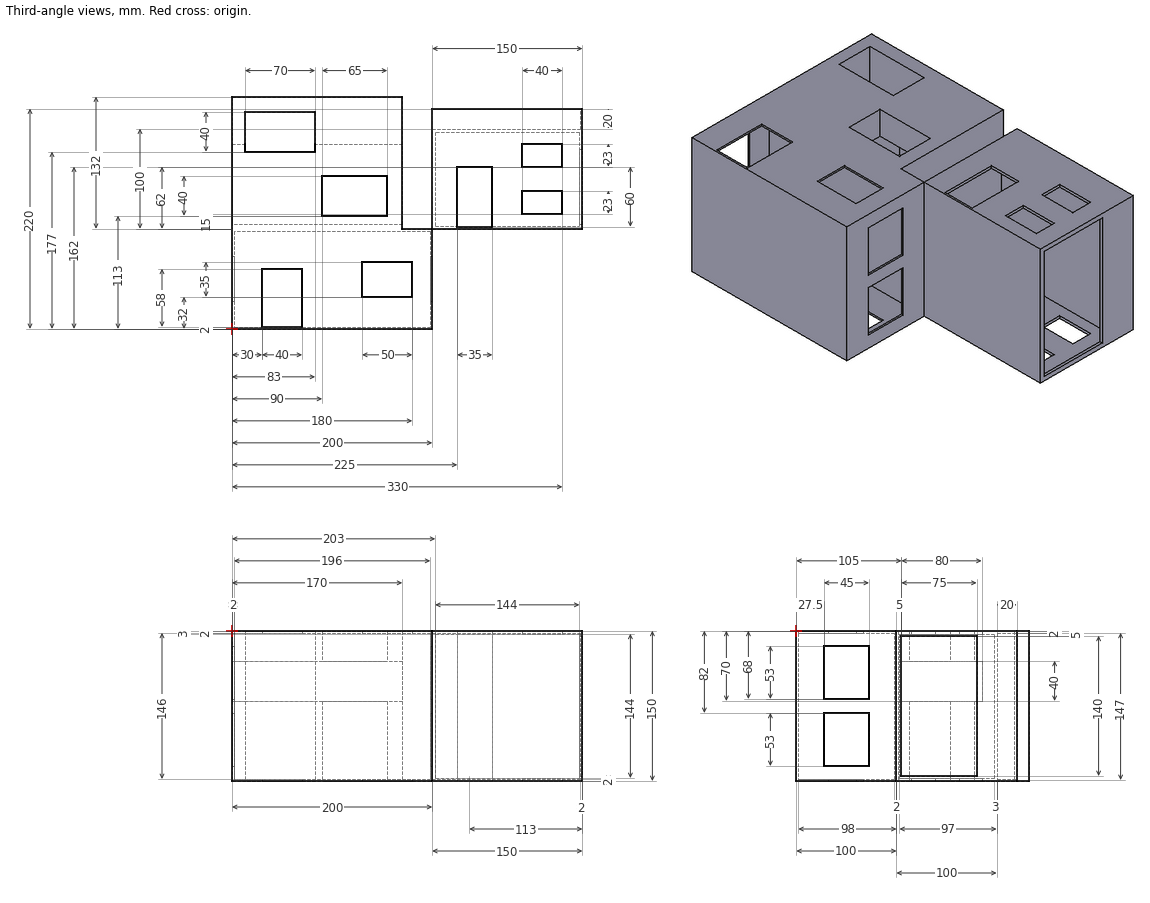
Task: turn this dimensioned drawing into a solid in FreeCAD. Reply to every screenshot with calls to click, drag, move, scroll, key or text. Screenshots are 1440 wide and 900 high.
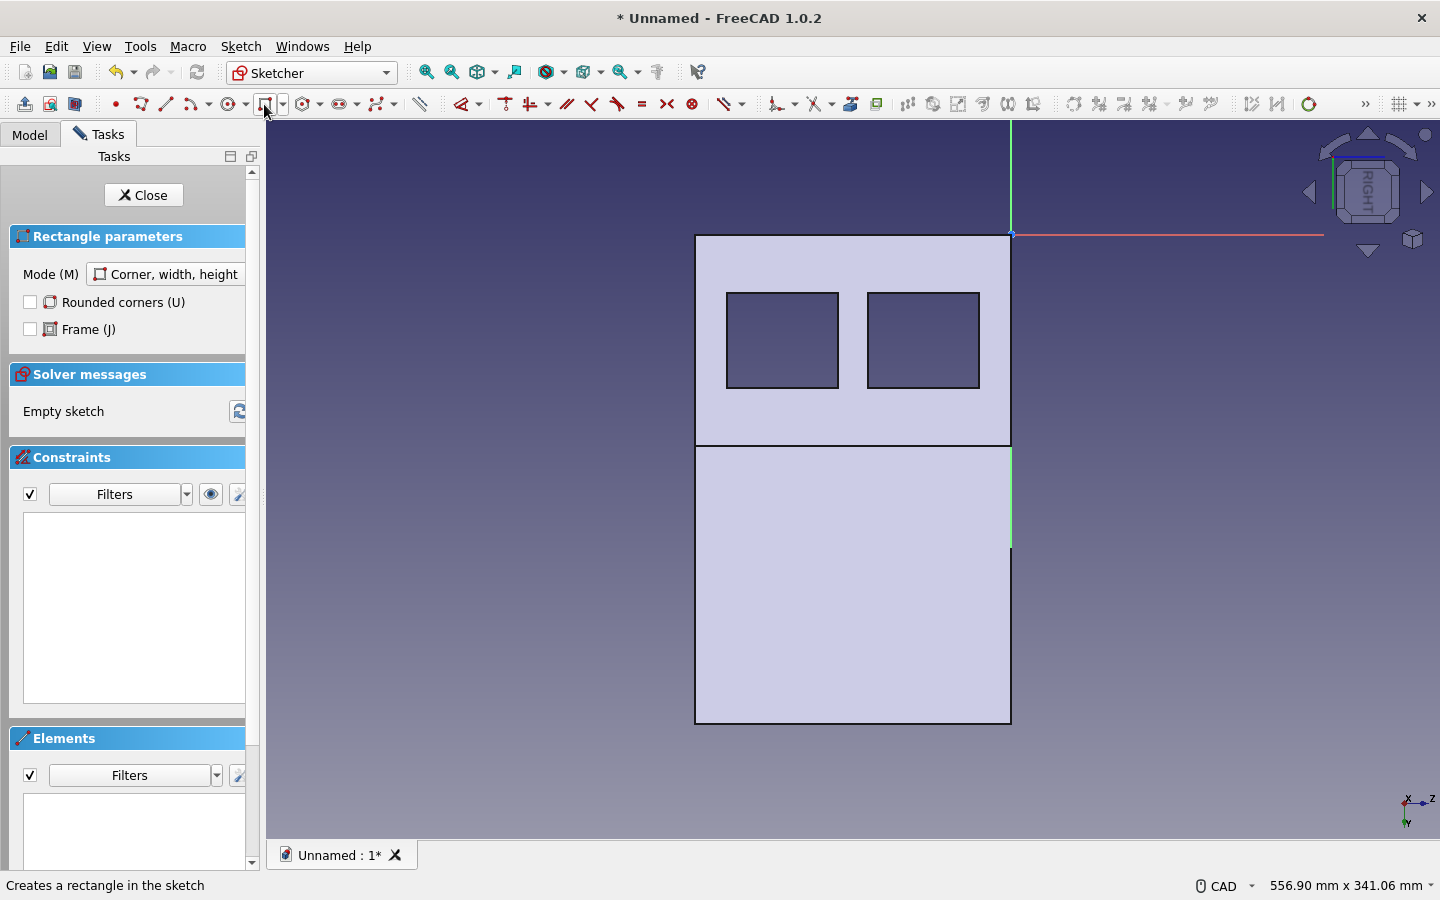
click(864, 456)
move(948, 625)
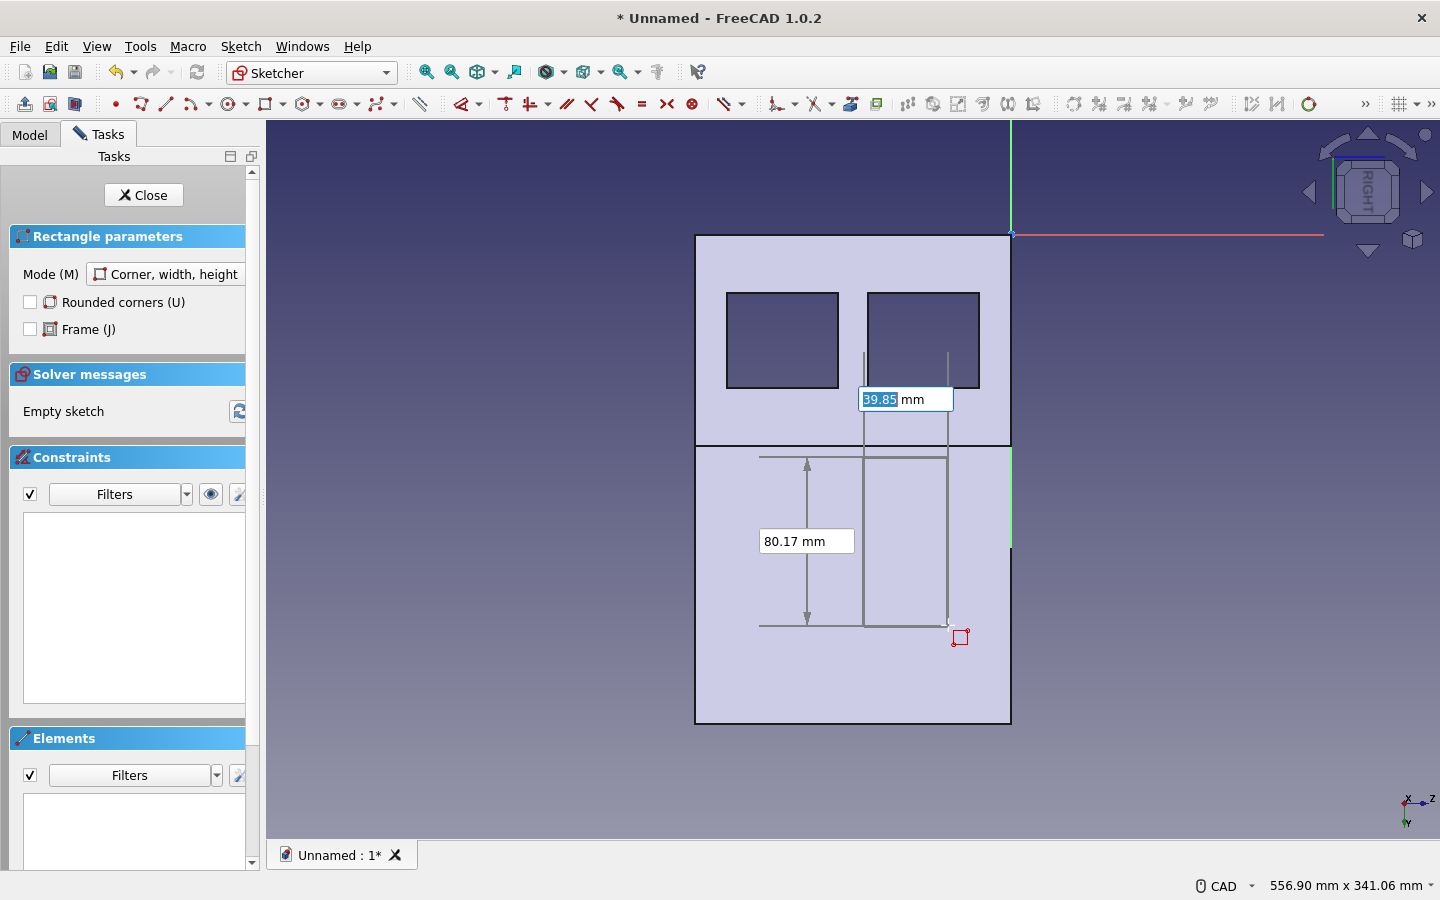
text(40)
key(Tab)
text(80)
key(Return)
key(Escape)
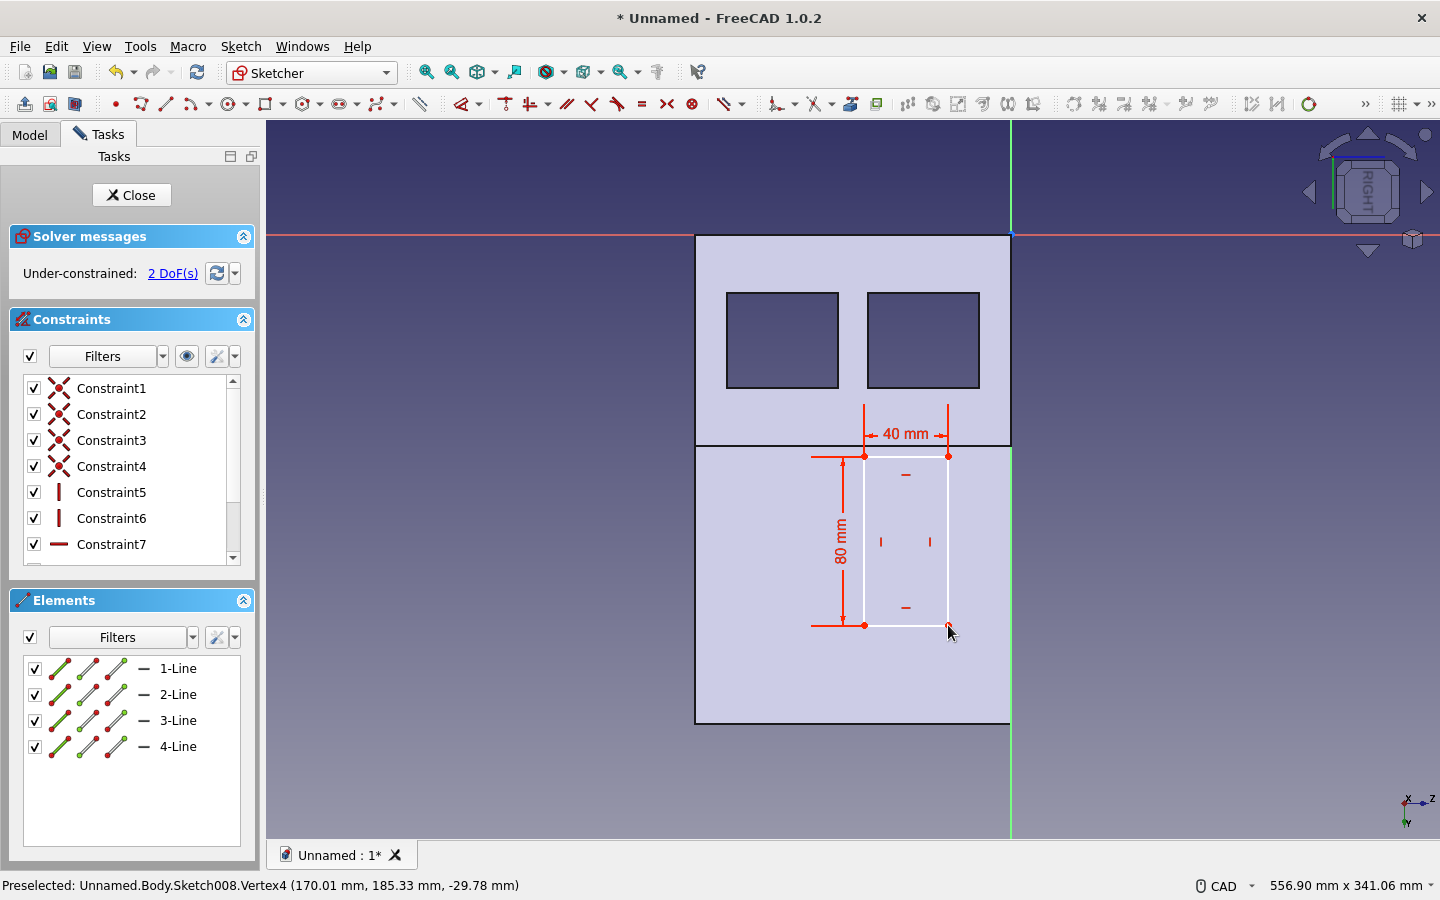
click(460, 104)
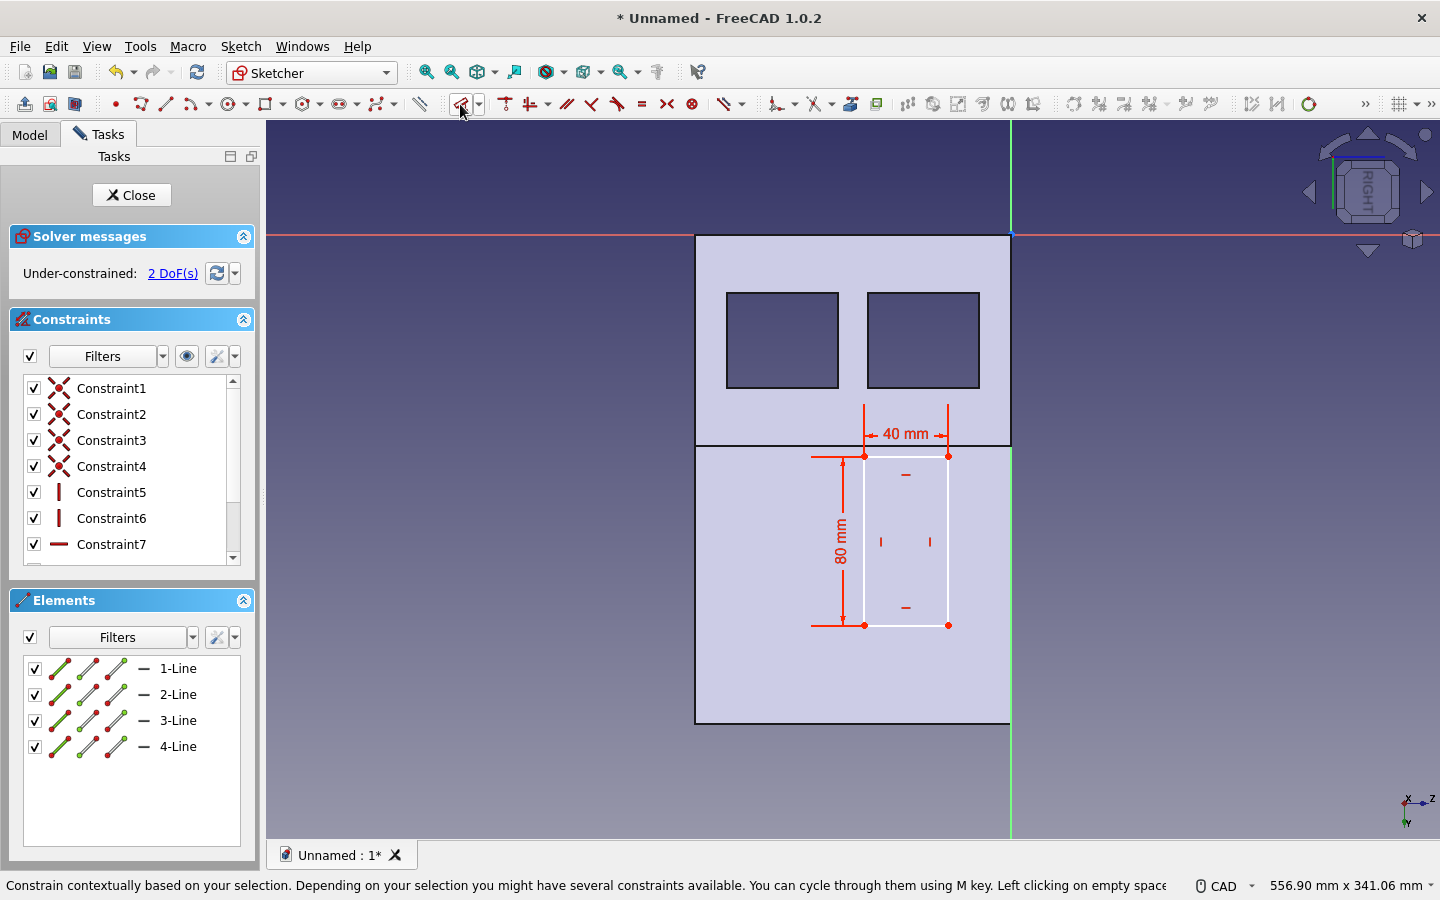
click(864, 457)
click(938, 201)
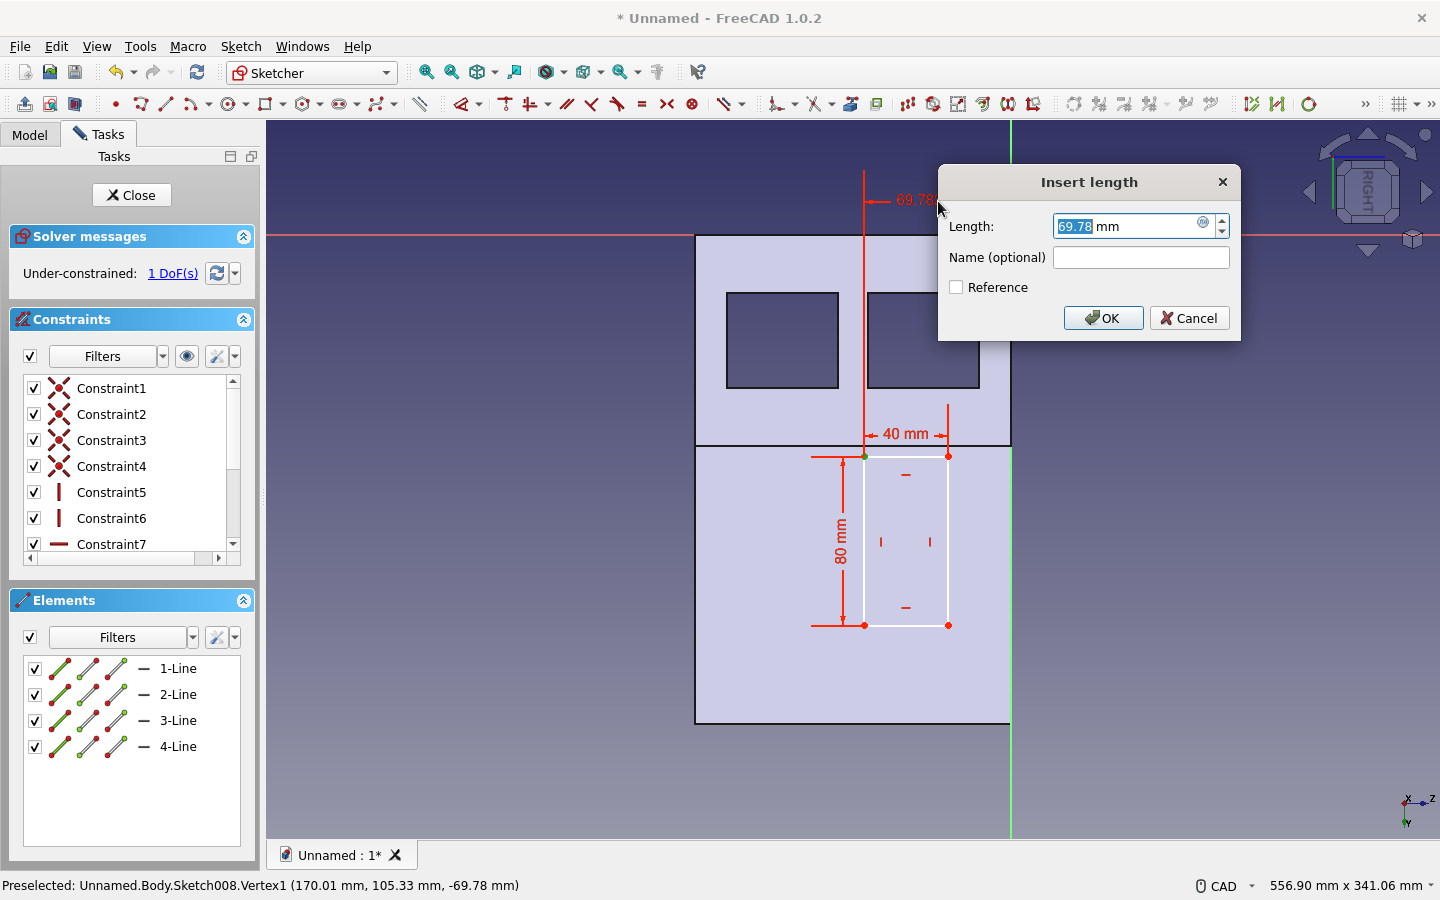
text(70)
key(Return)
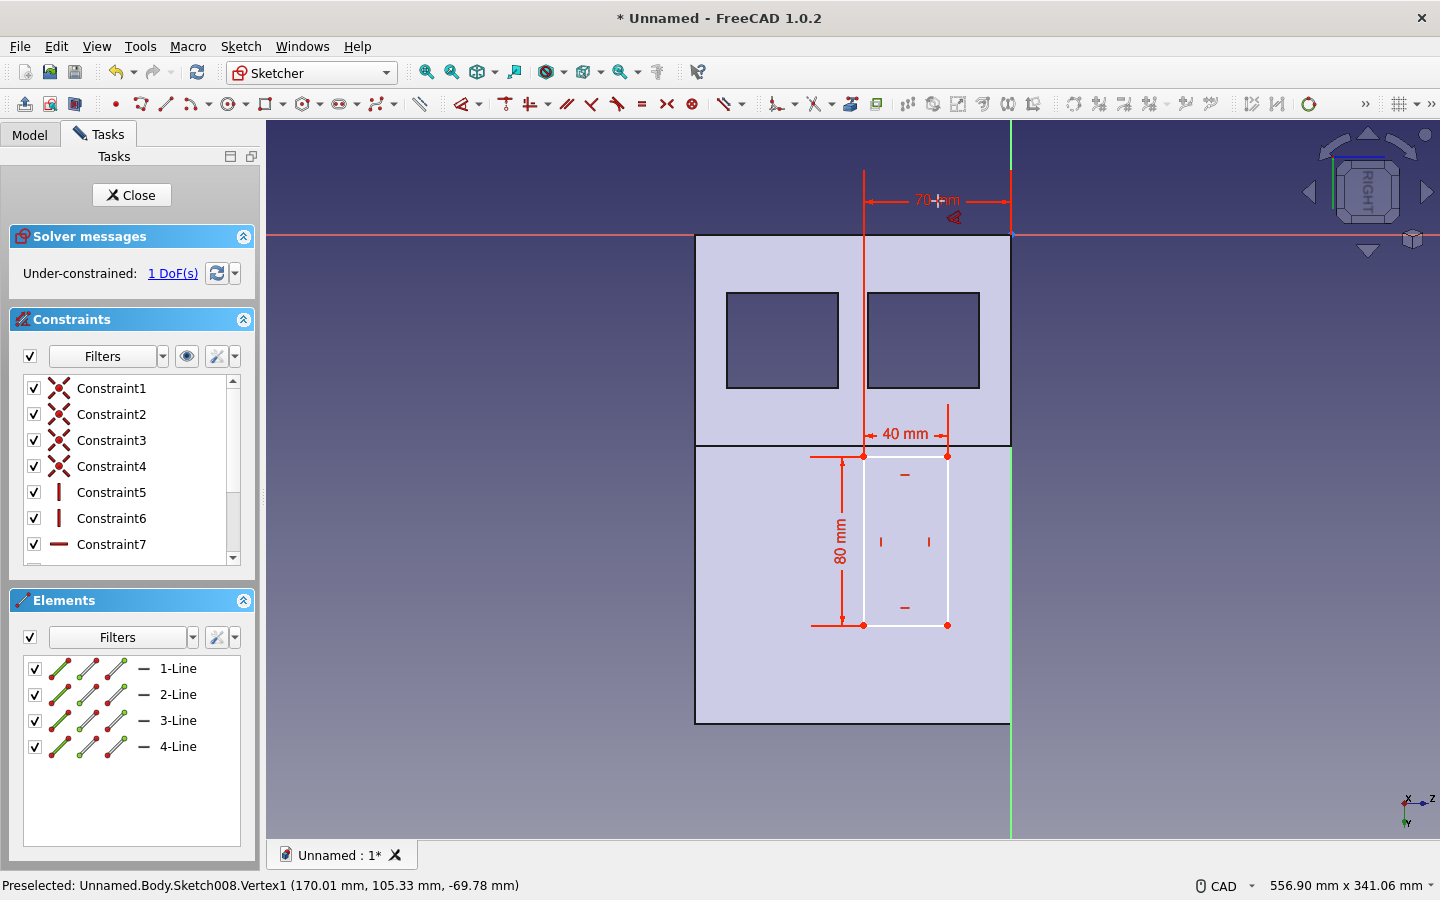
click(864, 457)
click(1045, 346)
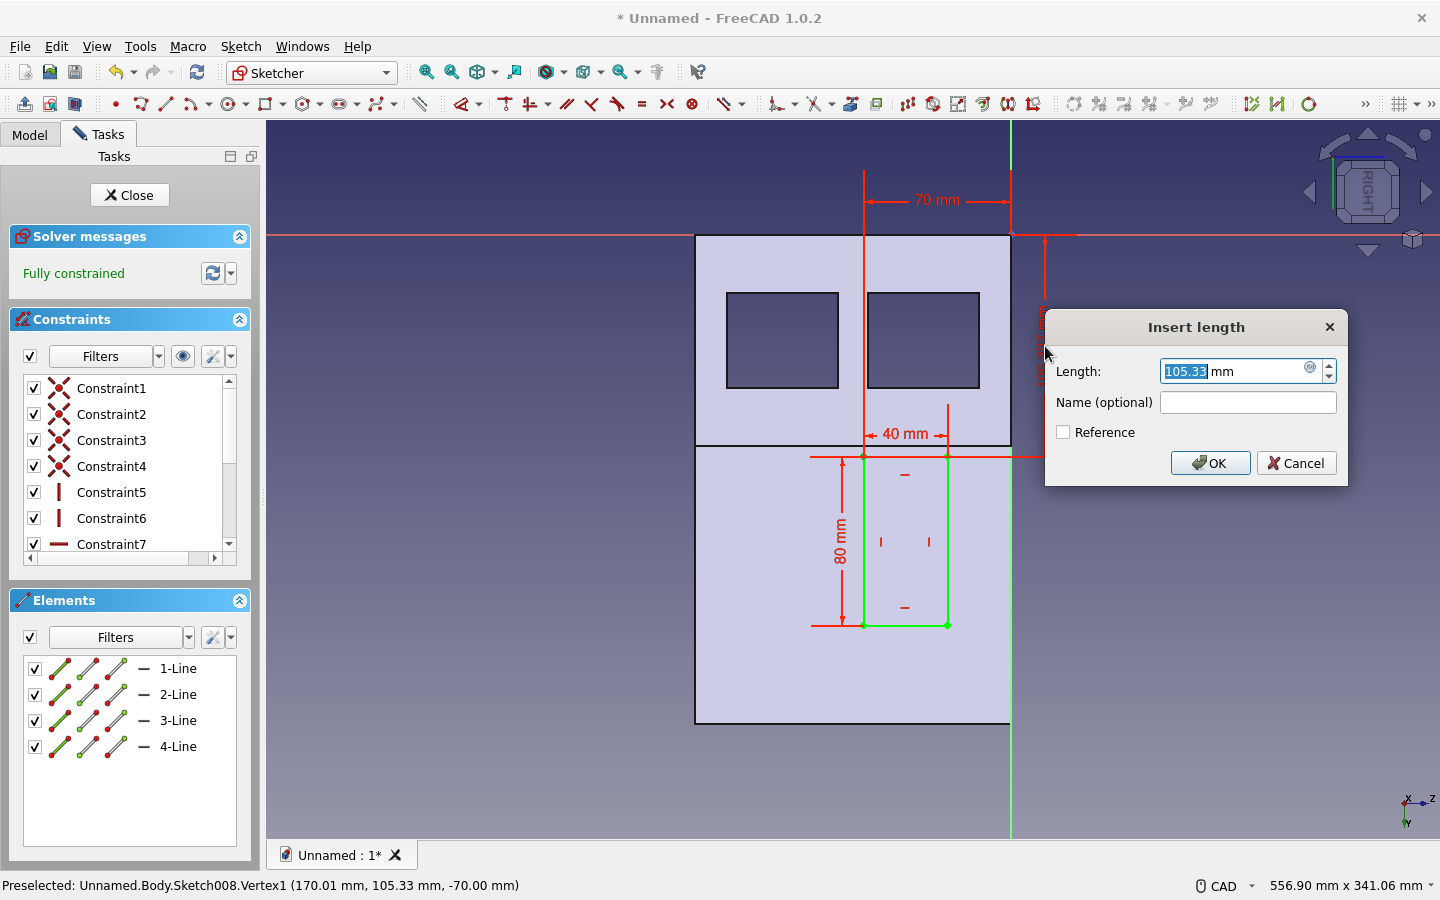
text(105)
key(Return)
key(Escape)